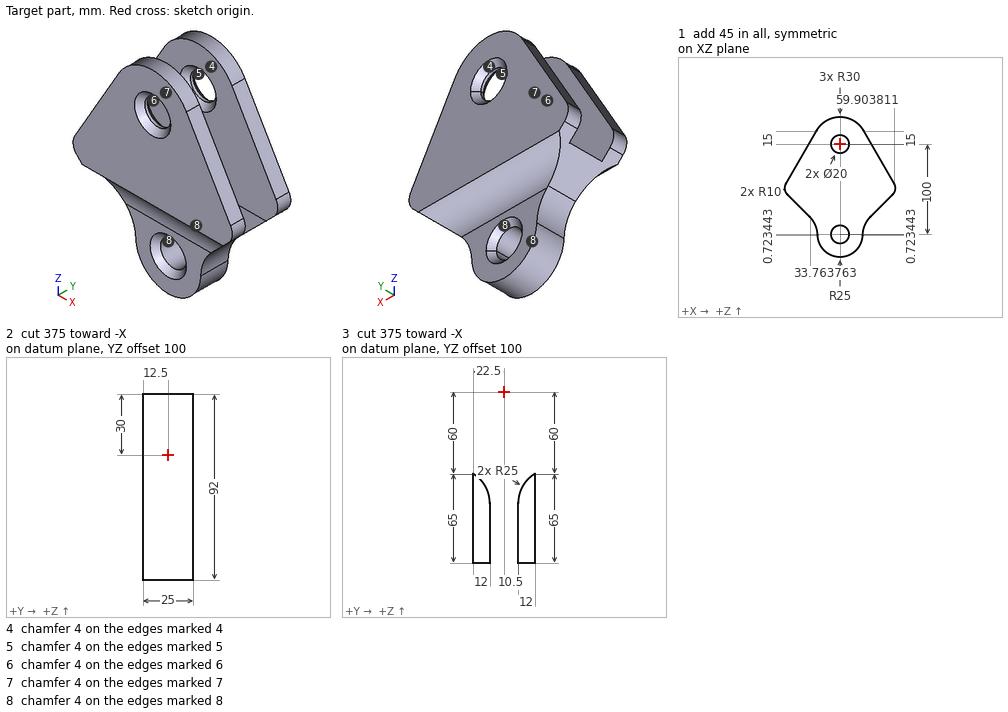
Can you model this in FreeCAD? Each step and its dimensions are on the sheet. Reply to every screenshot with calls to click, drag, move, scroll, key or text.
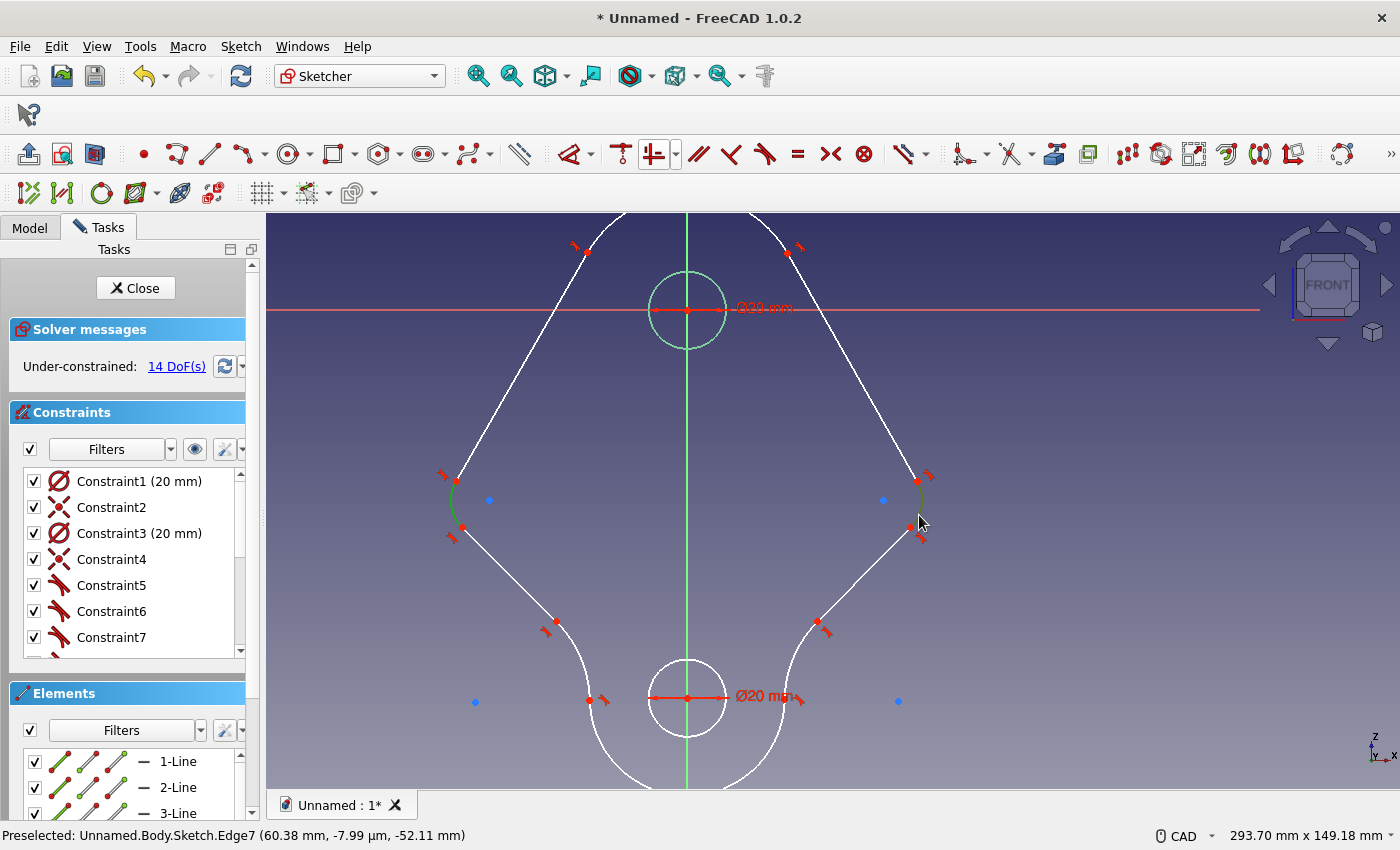
click(798, 154)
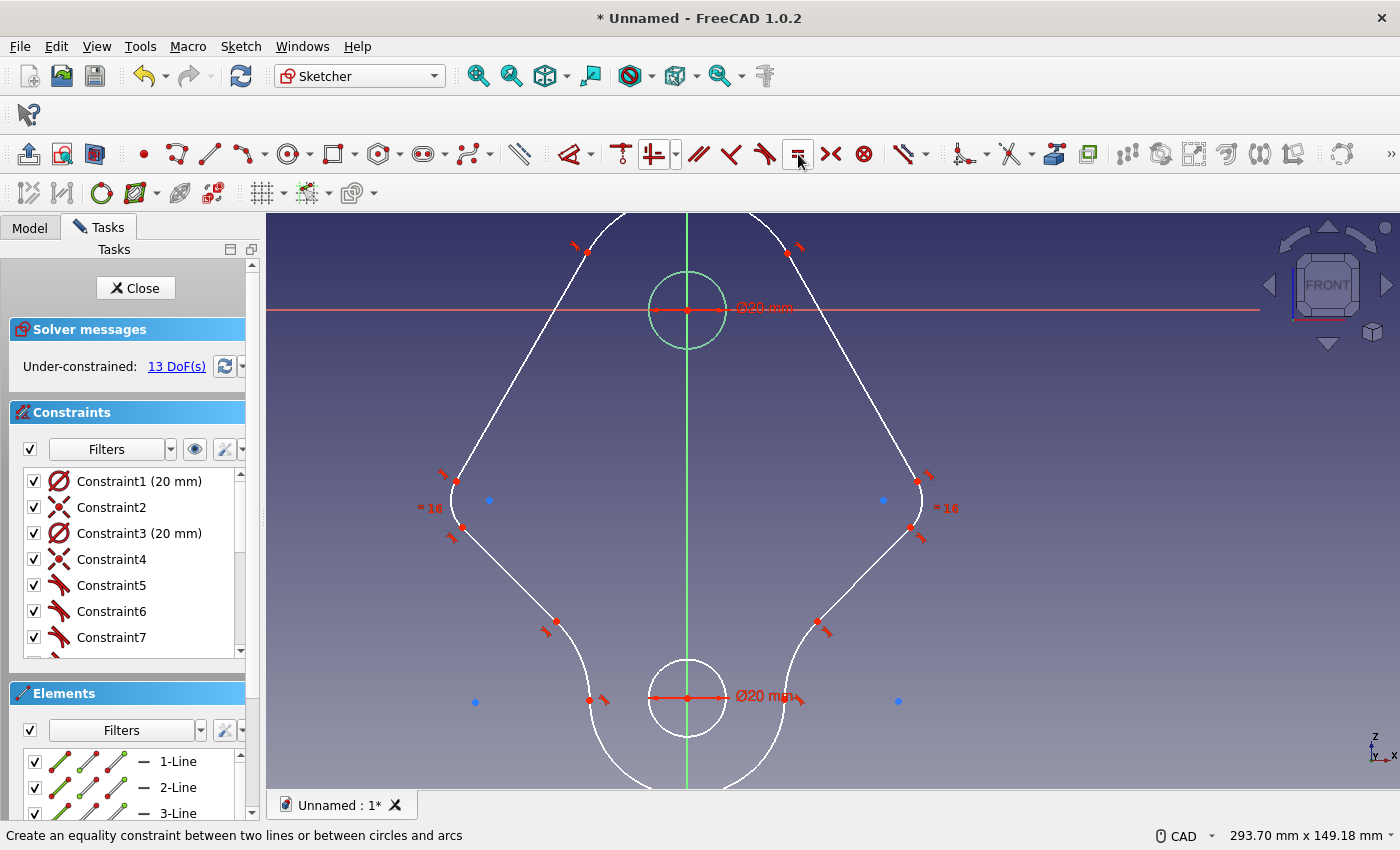
scroll(921, 516, down, 2)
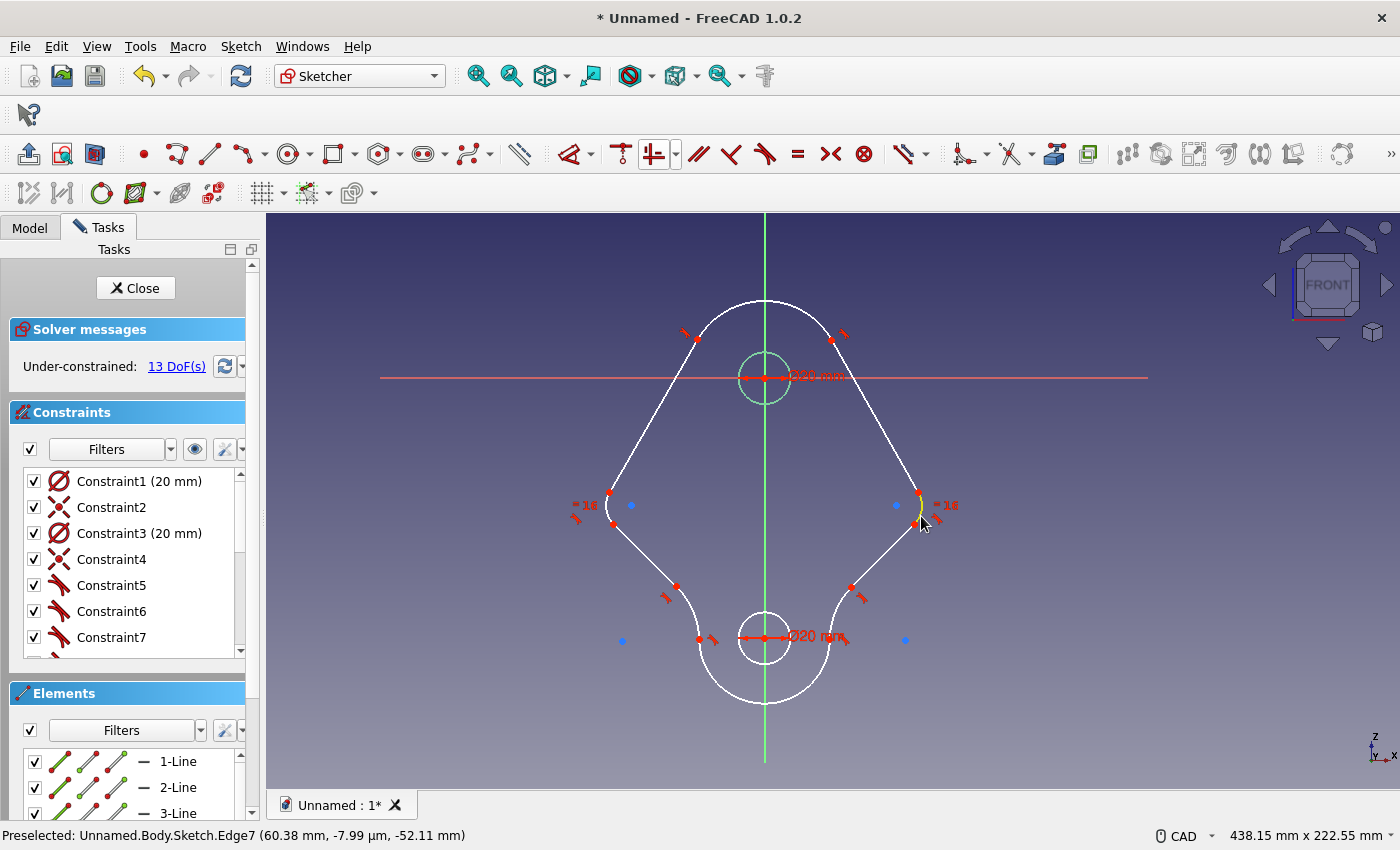
click(796, 308)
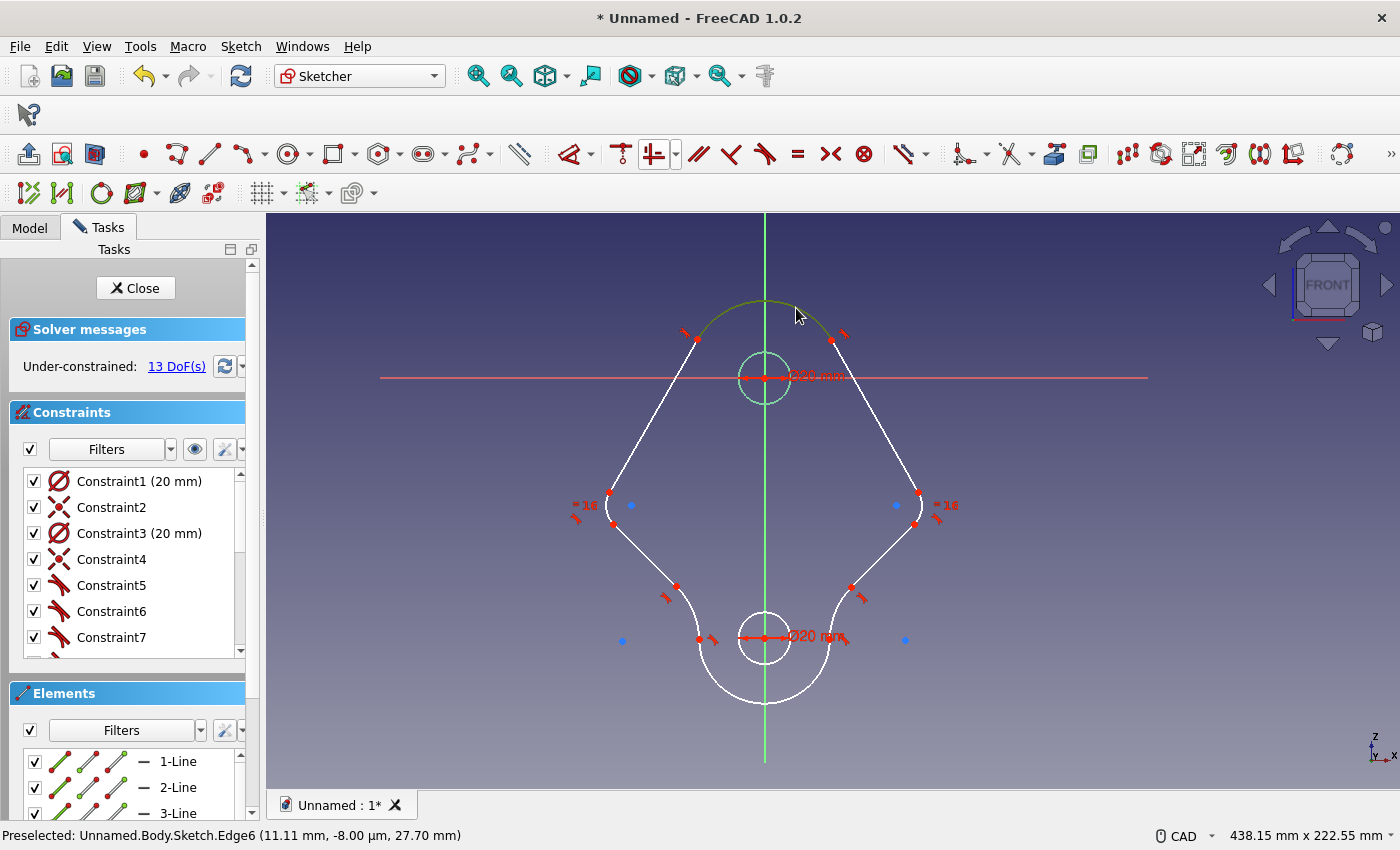
click(841, 601)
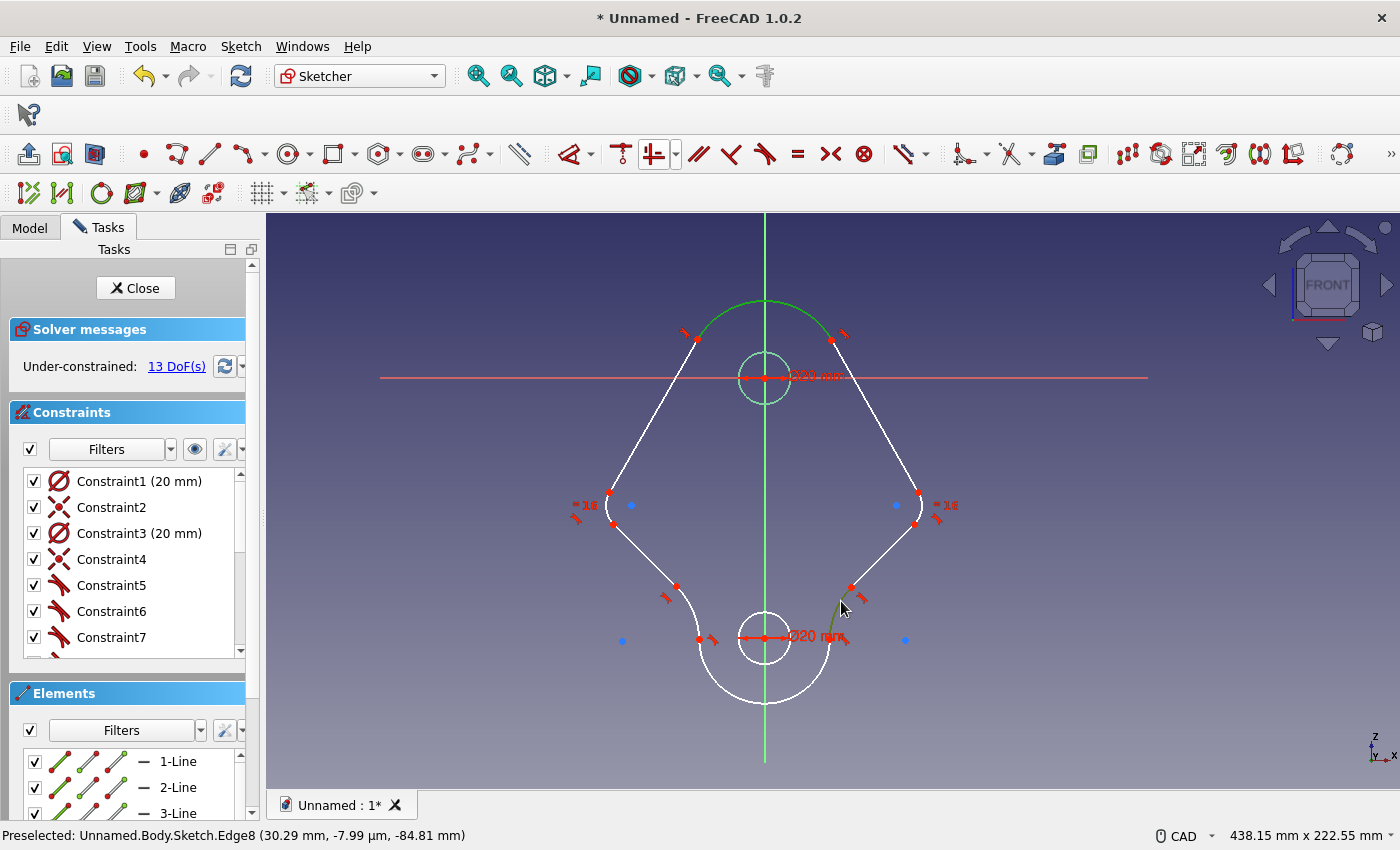
click(697, 622)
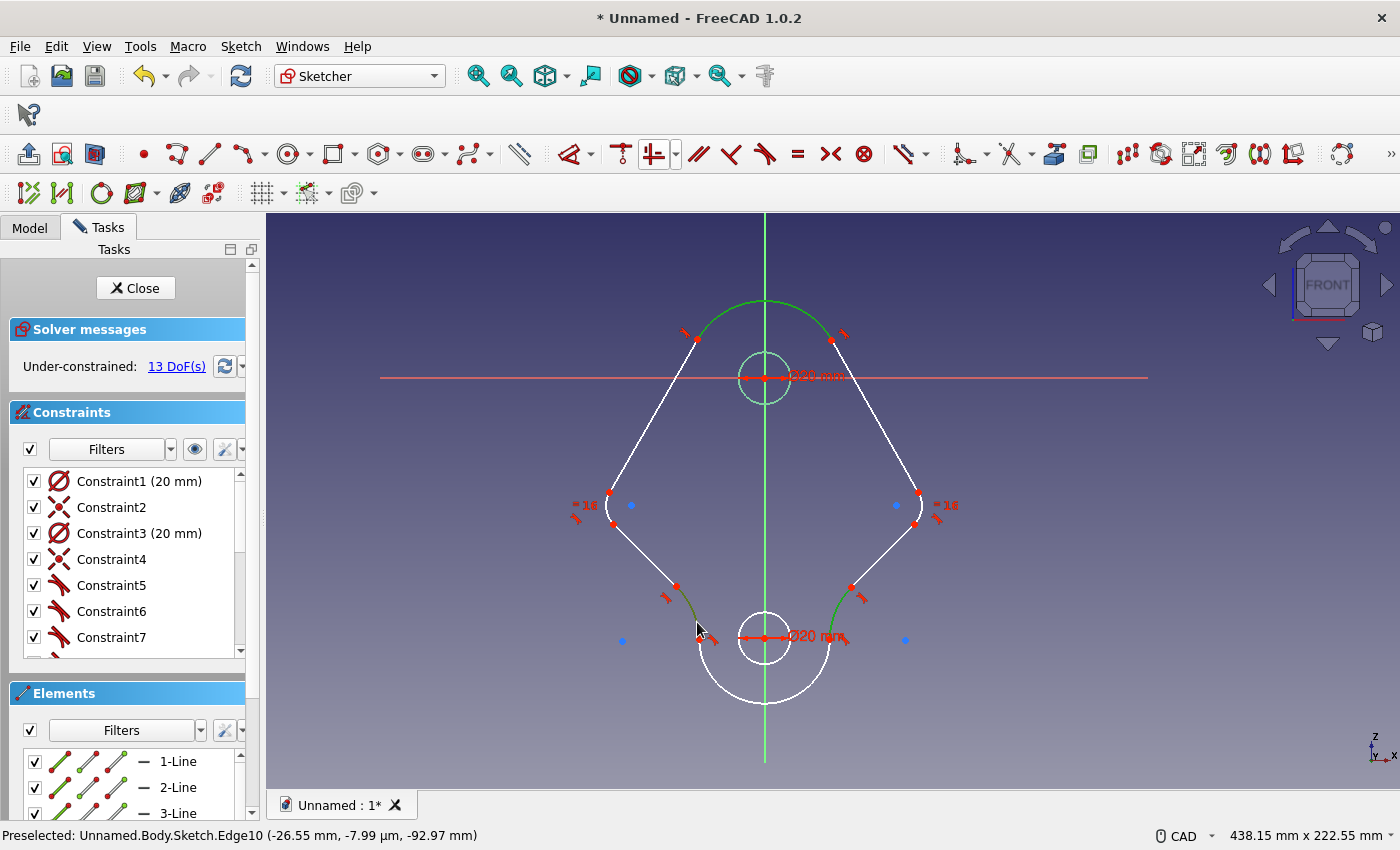
click(798, 154)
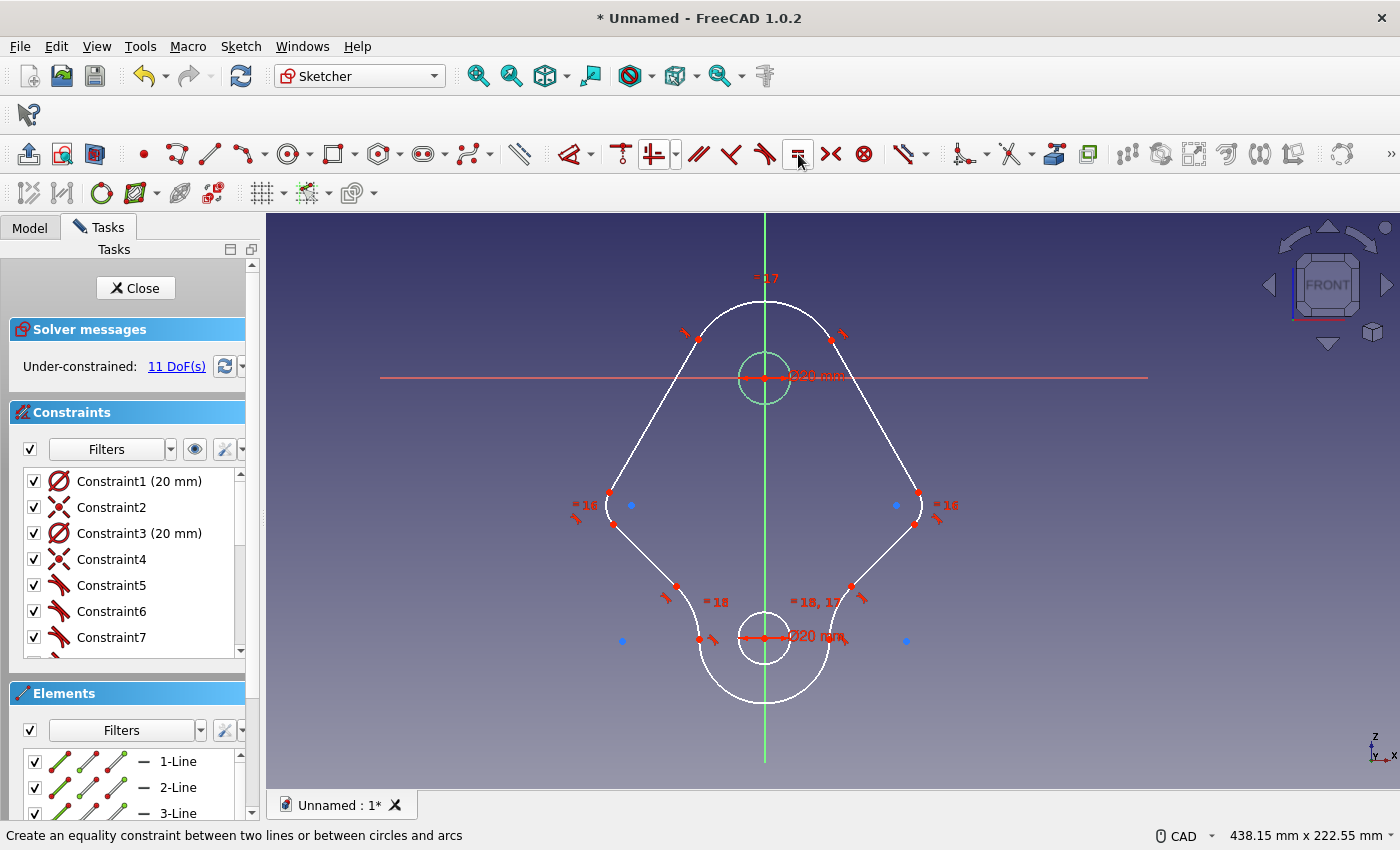
click(764, 638)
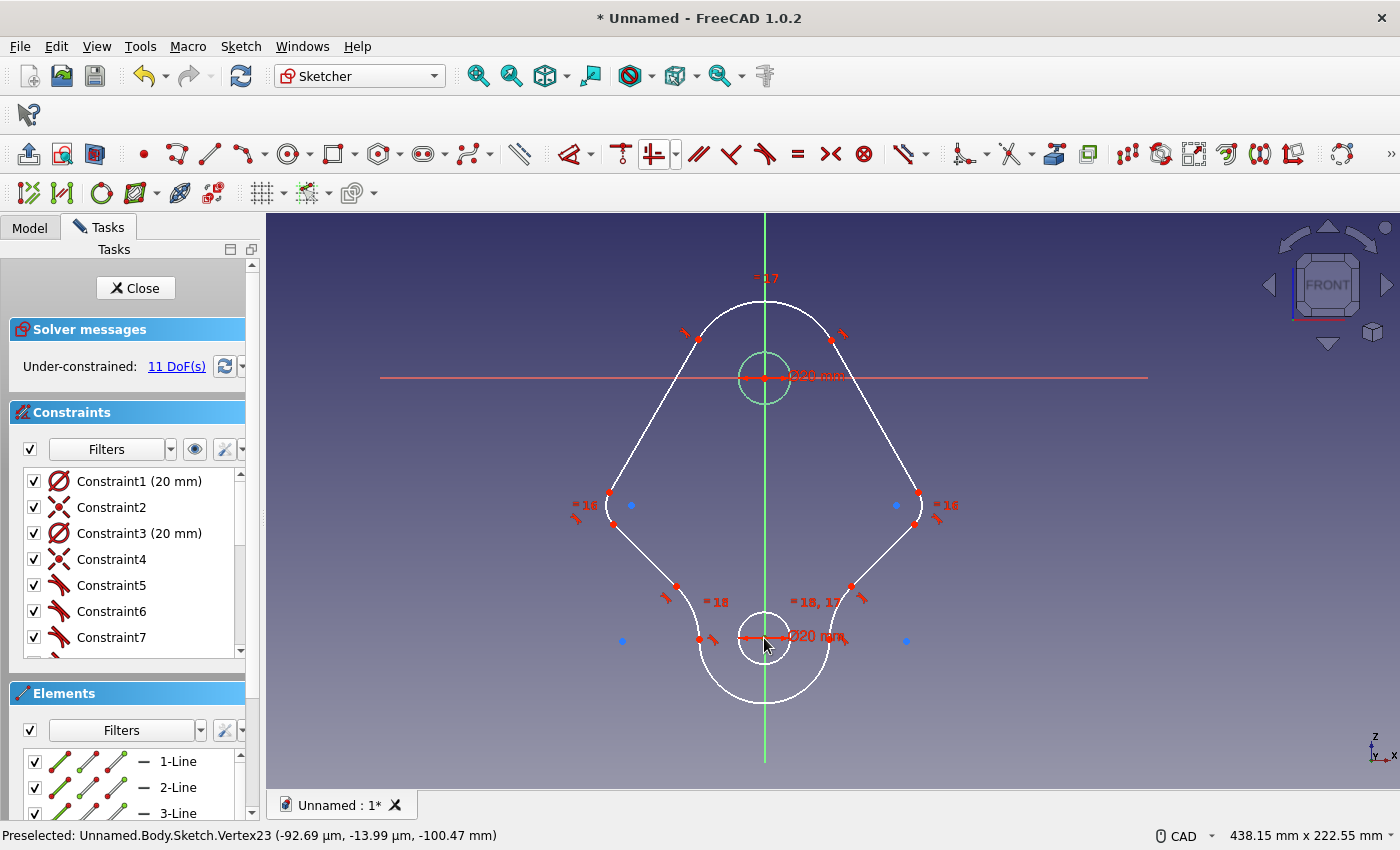
click(765, 575)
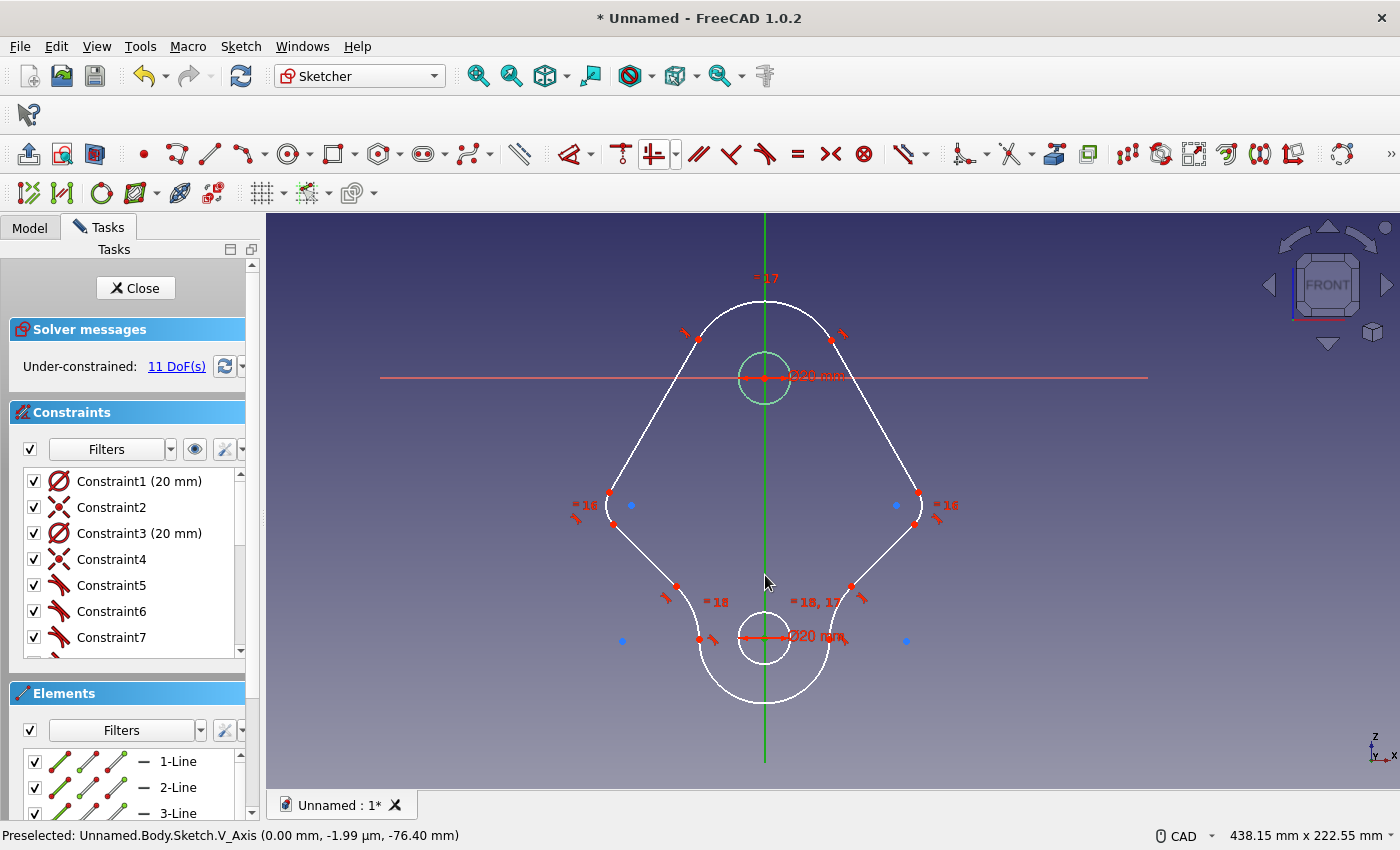
click(621, 154)